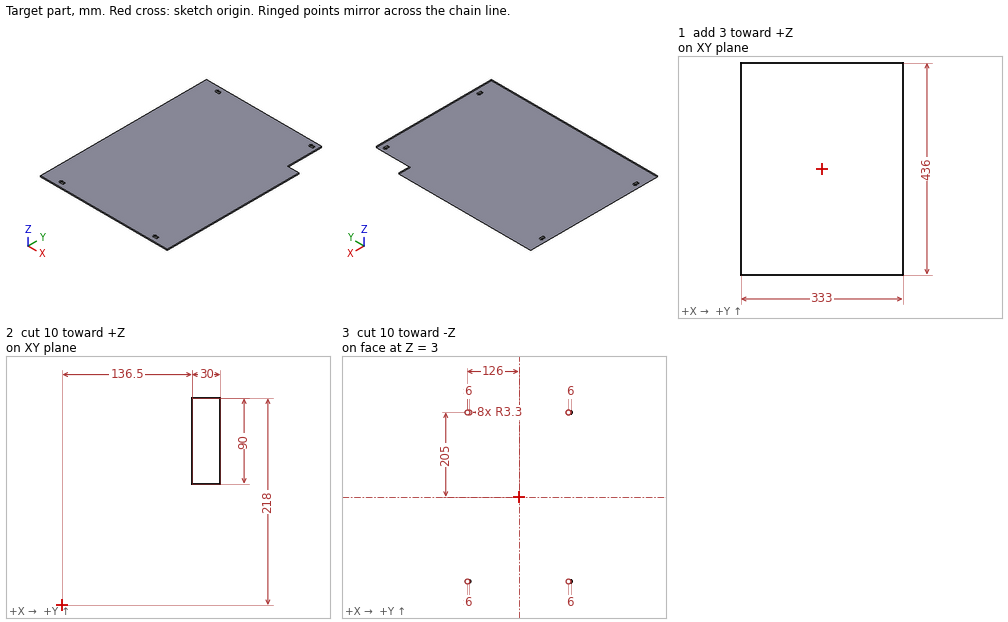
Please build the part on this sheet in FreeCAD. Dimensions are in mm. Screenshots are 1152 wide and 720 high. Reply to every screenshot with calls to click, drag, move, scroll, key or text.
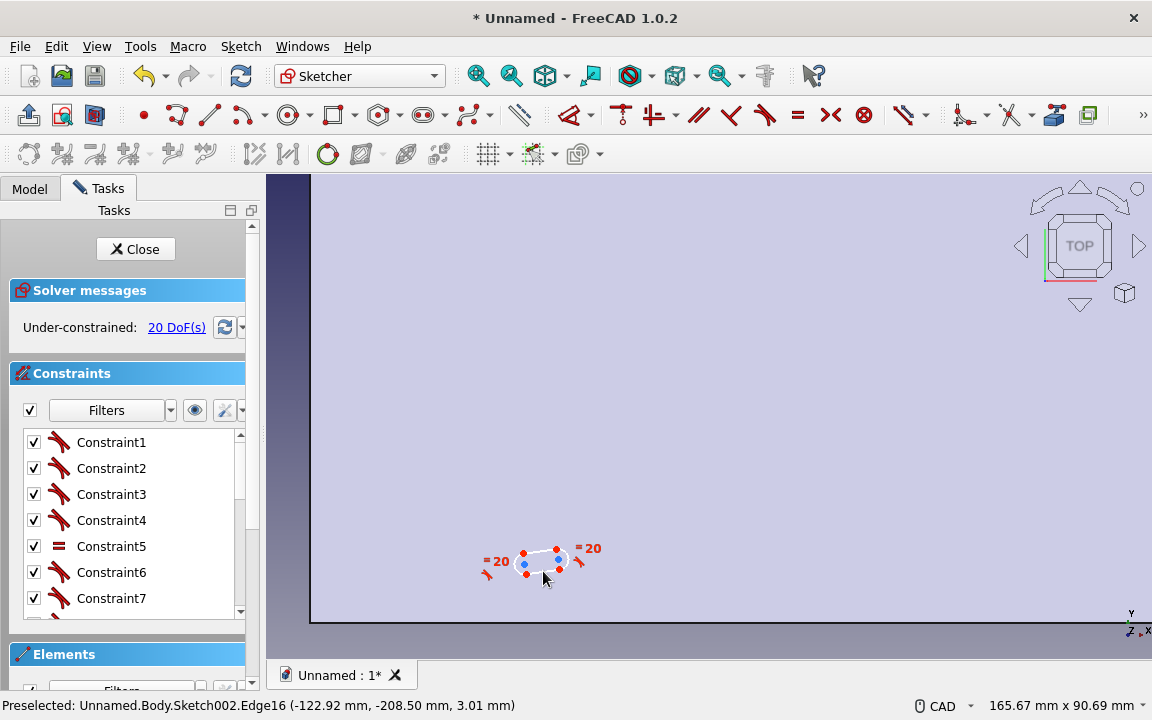
scroll(553, 567, down, 10)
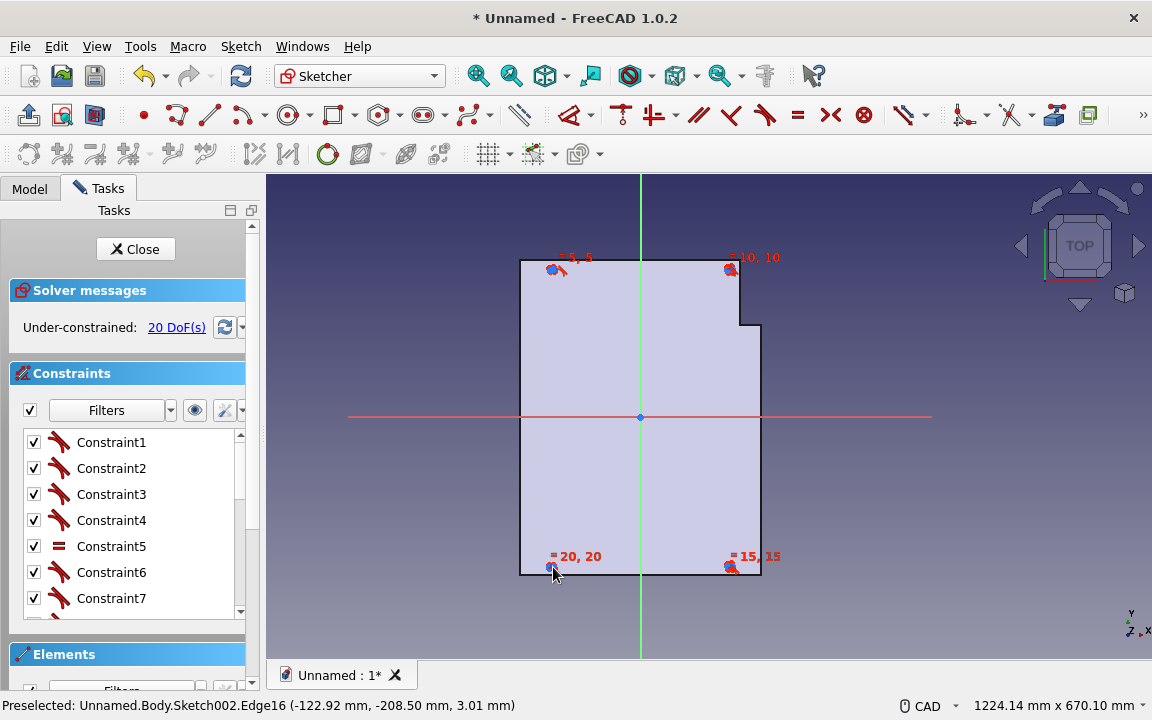
scroll(551, 268, up, 11)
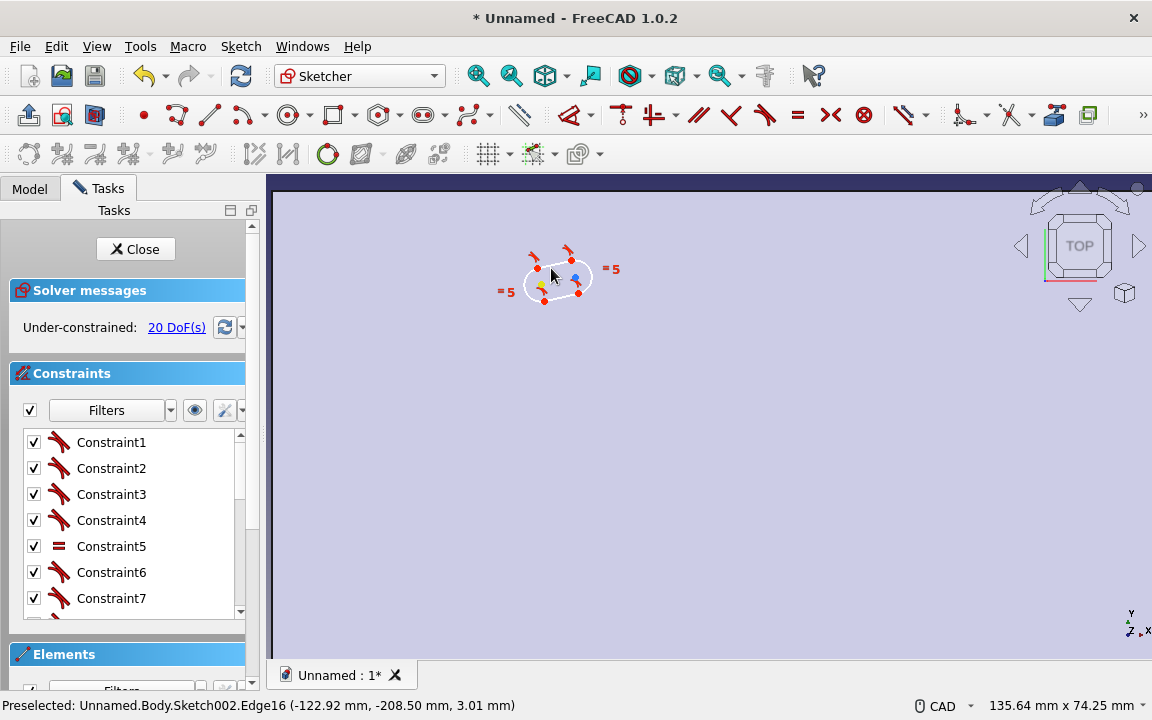
click(551, 265)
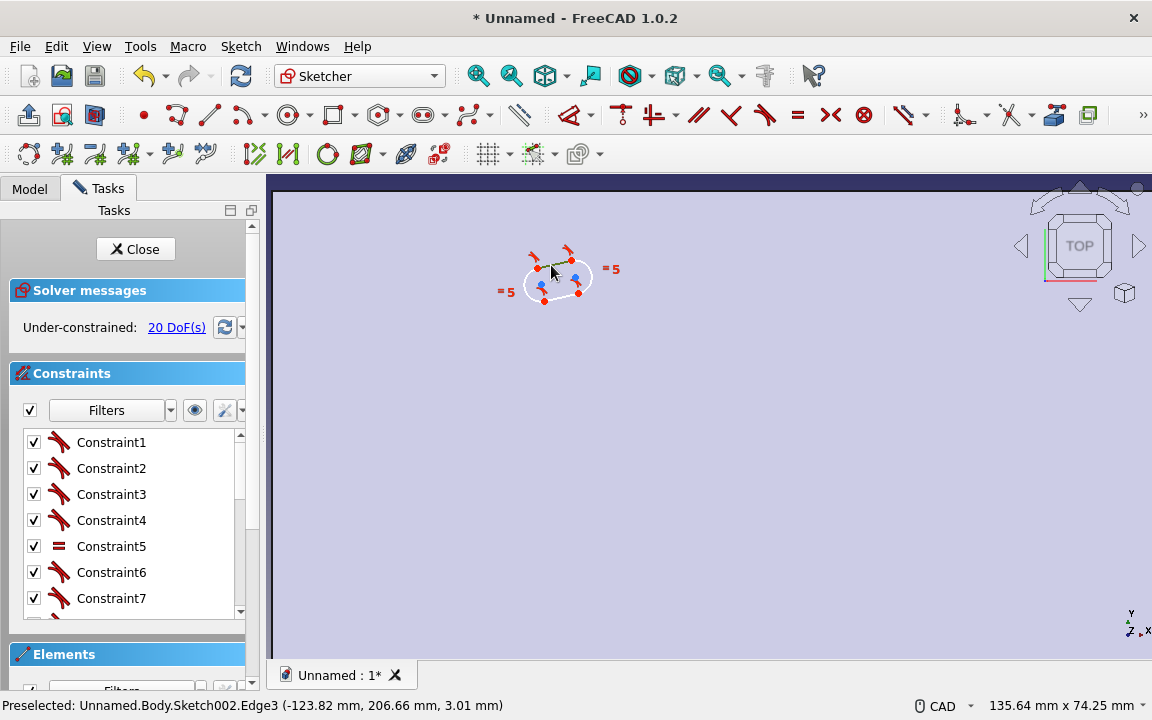
key(h)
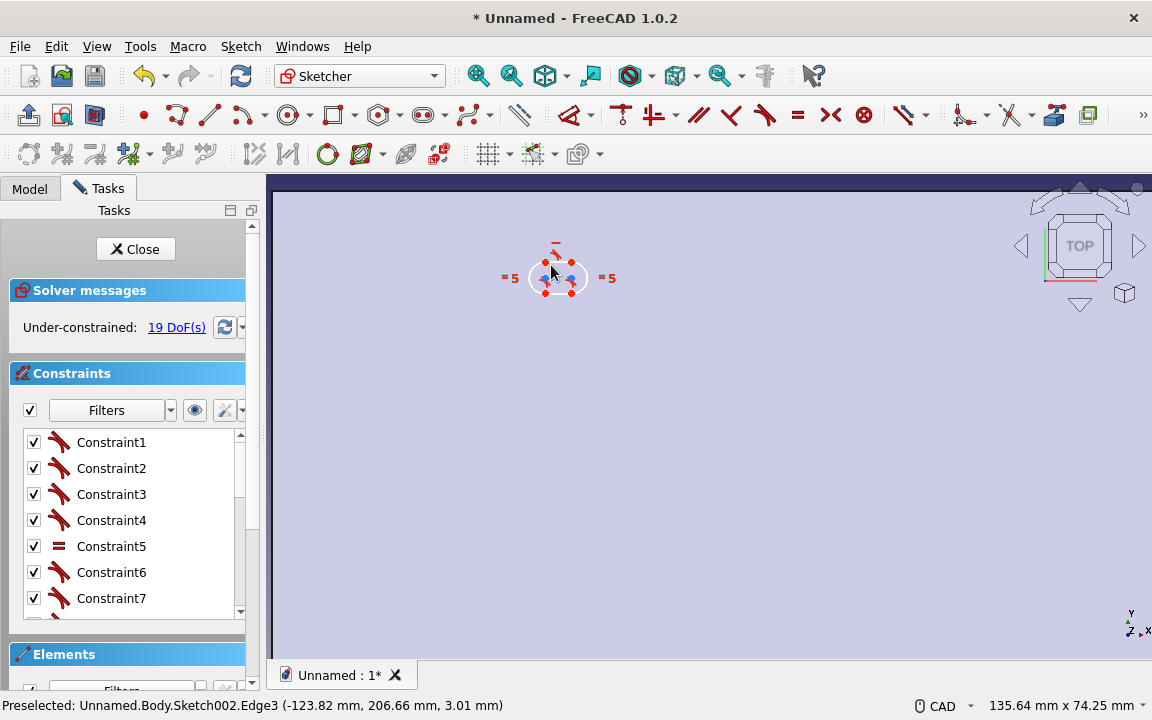
scroll(551, 267, down, 11)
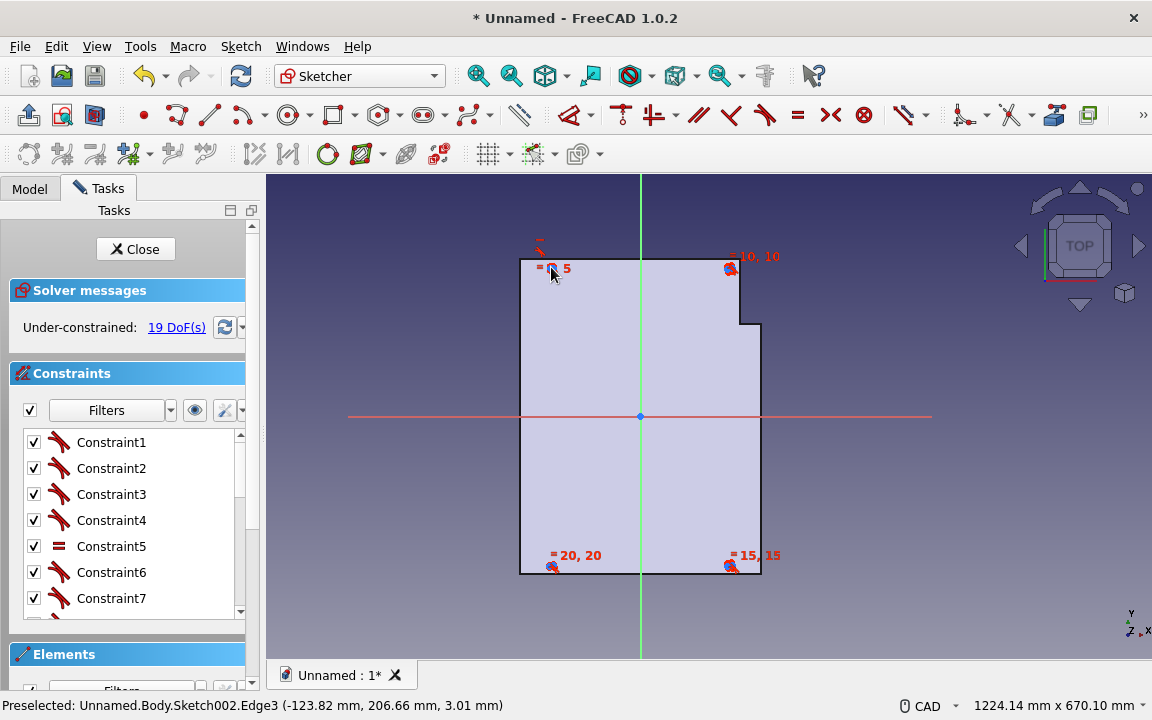
scroll(729, 266, up, 12)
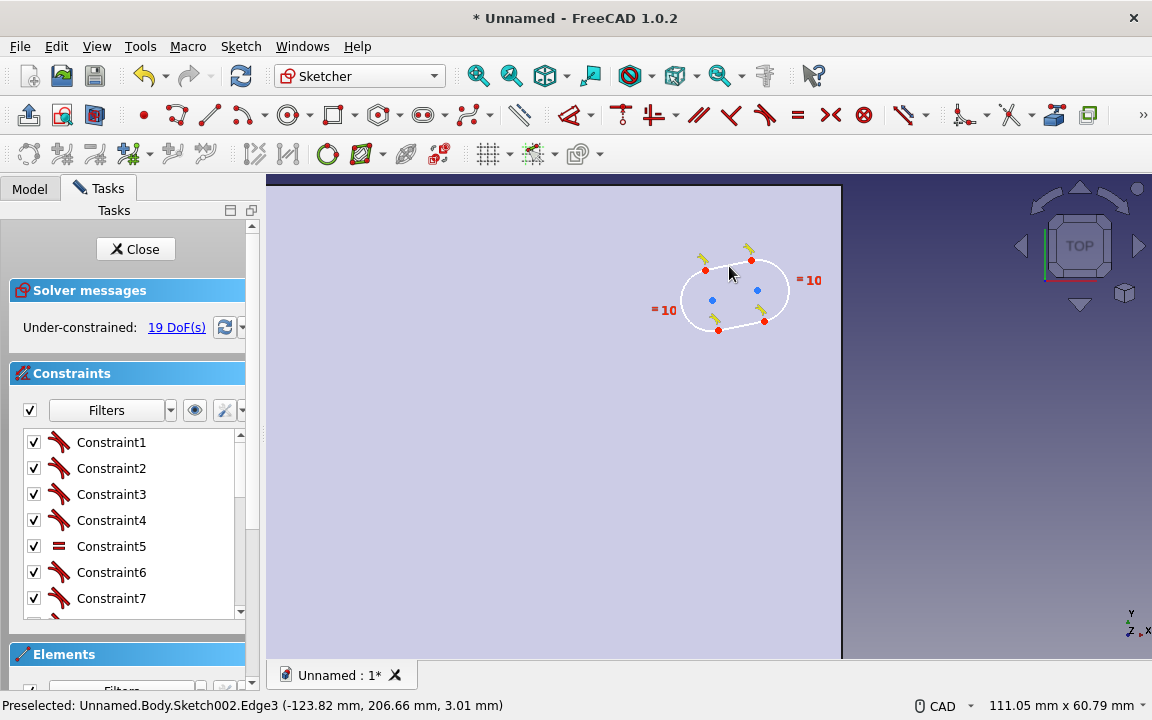
click(720, 267)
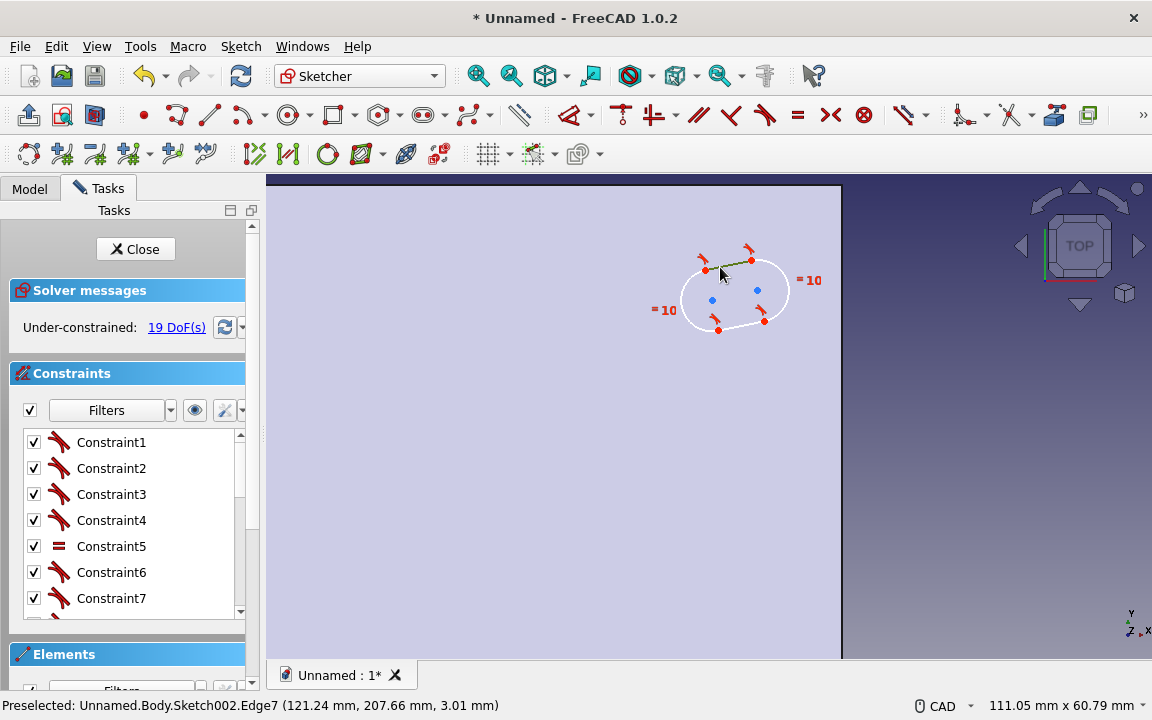
click(676, 116)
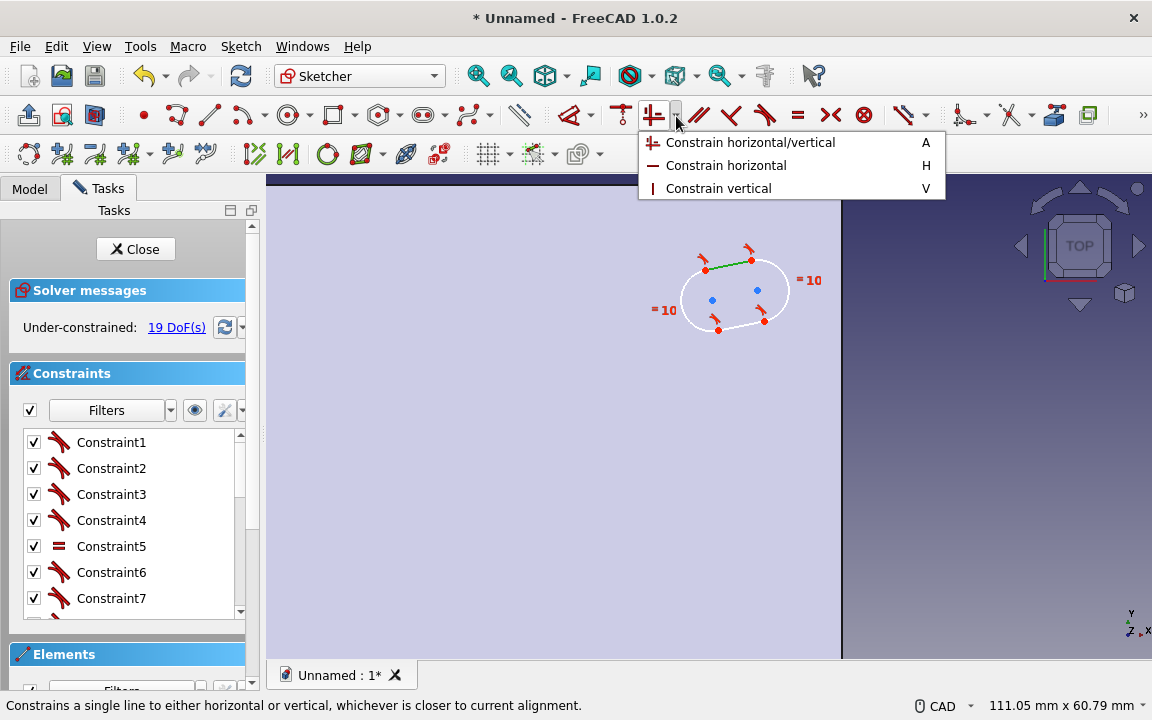
click(792, 166)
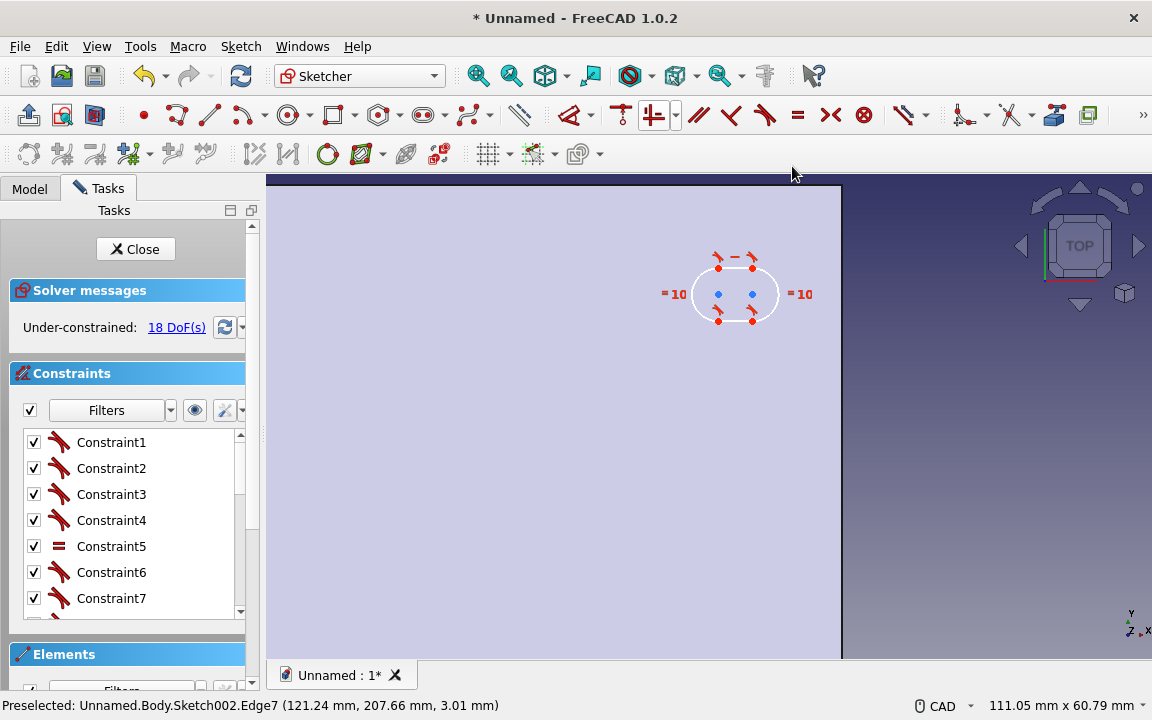
scroll(729, 266, down, 12)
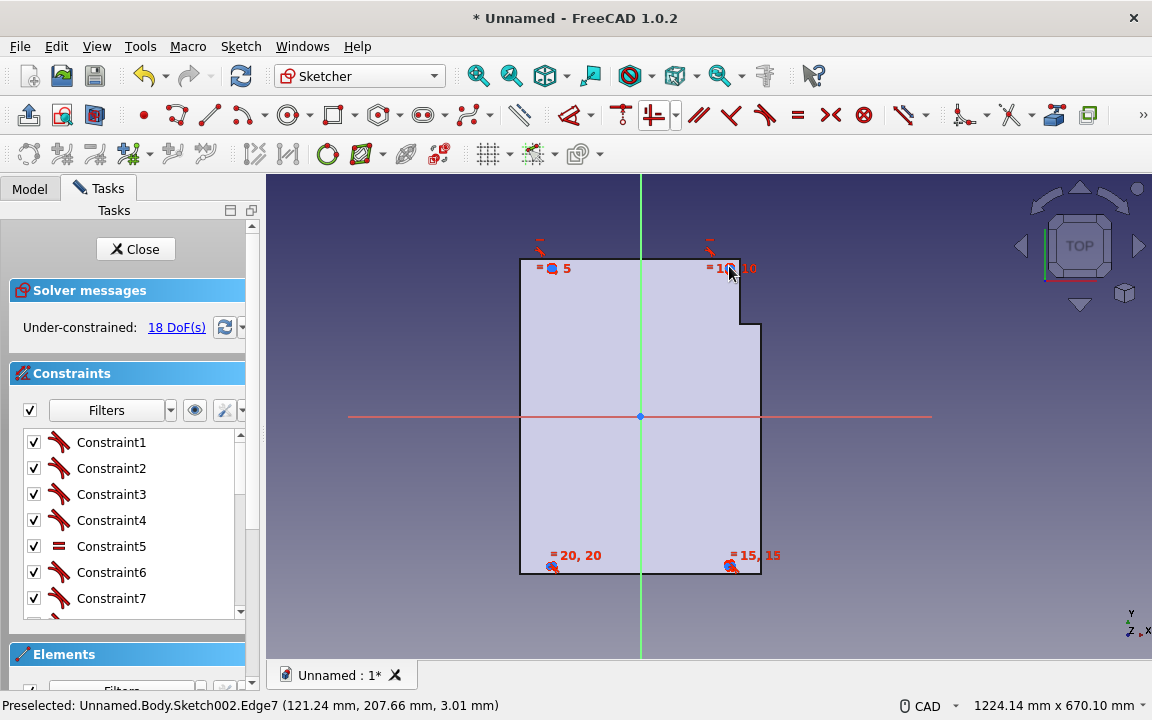
scroll(729, 563, up, 12)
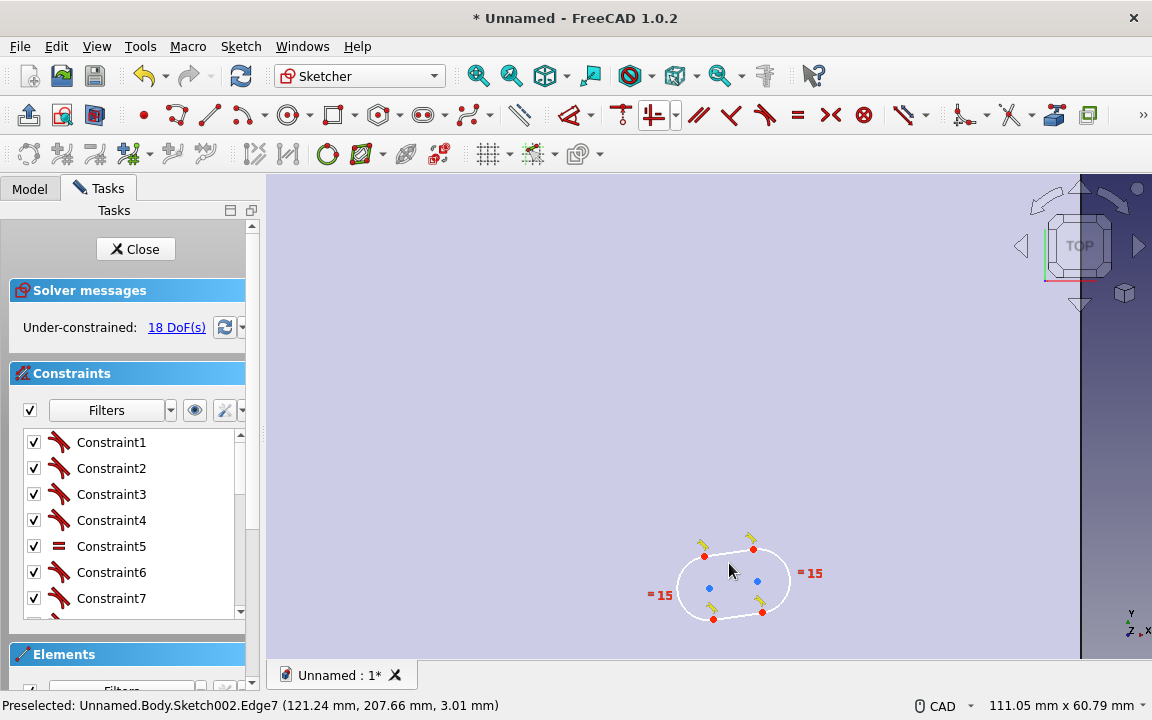
click(719, 554)